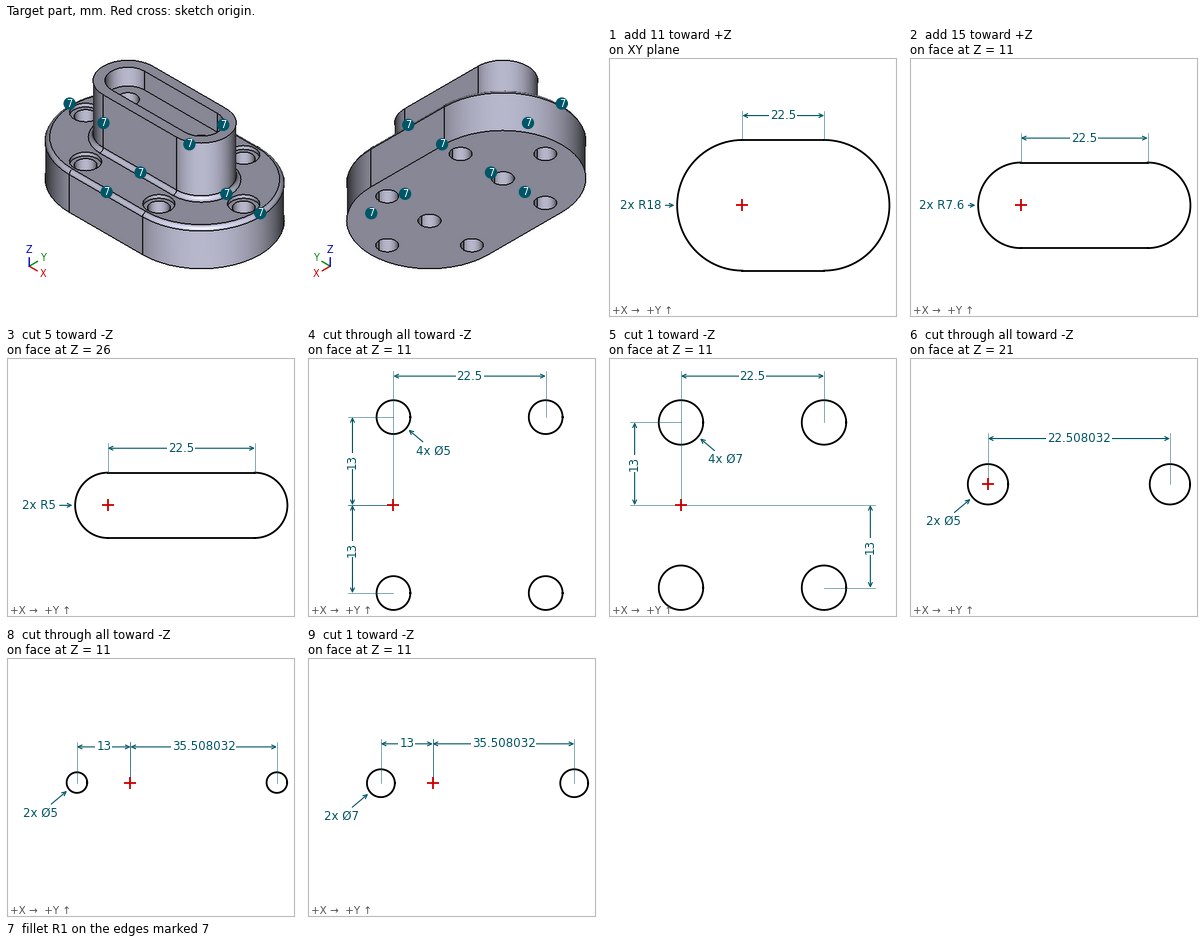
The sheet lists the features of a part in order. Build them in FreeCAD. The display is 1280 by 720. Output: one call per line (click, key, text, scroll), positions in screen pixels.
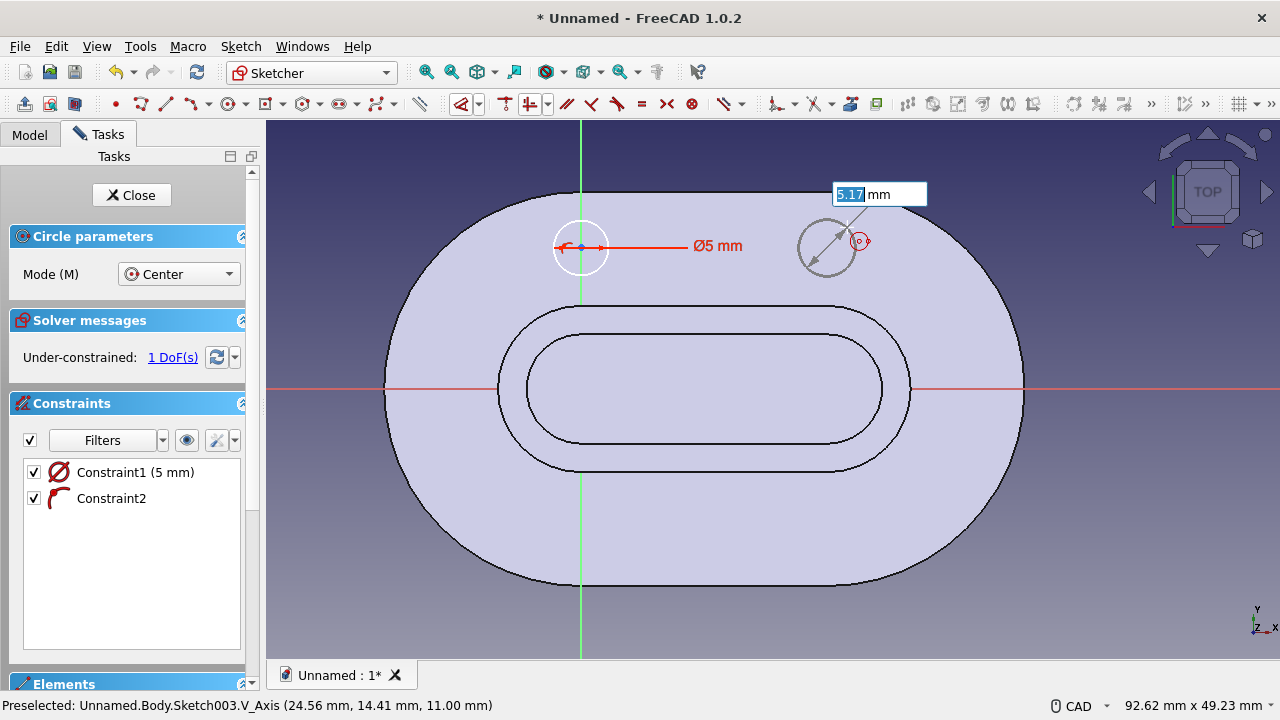
text(5)
key(Return)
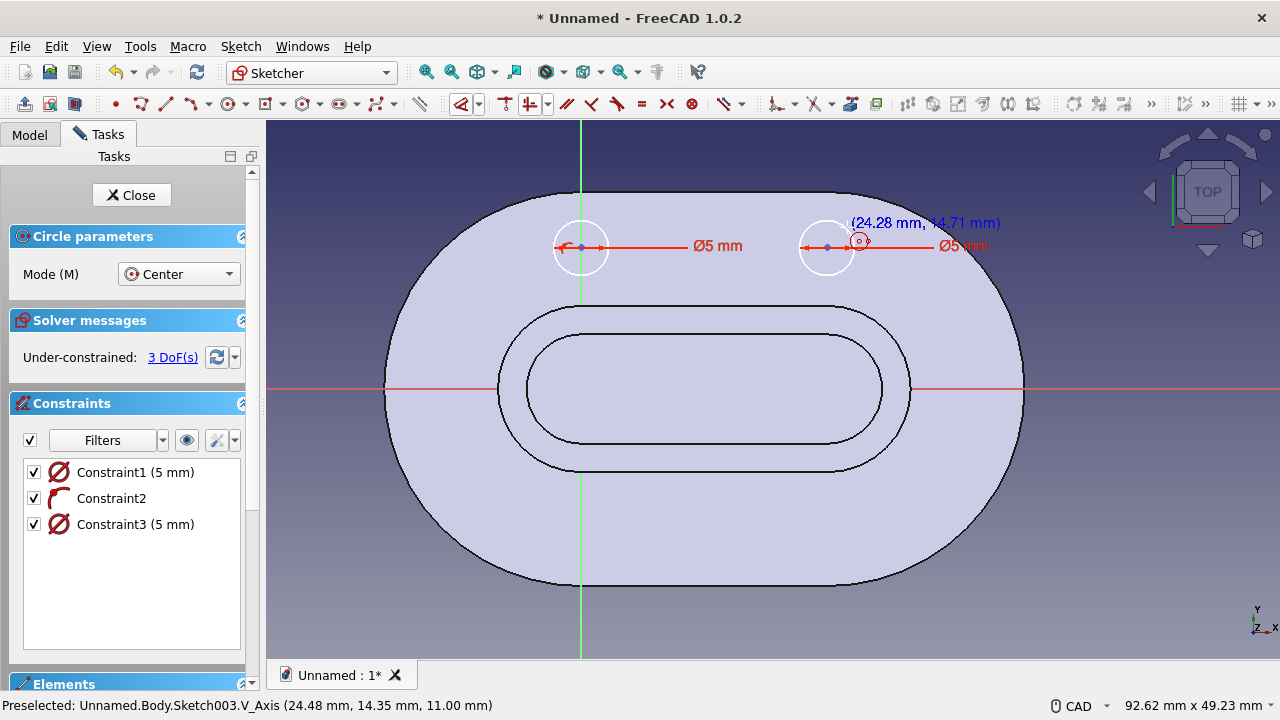
click(581, 531)
move(601, 512)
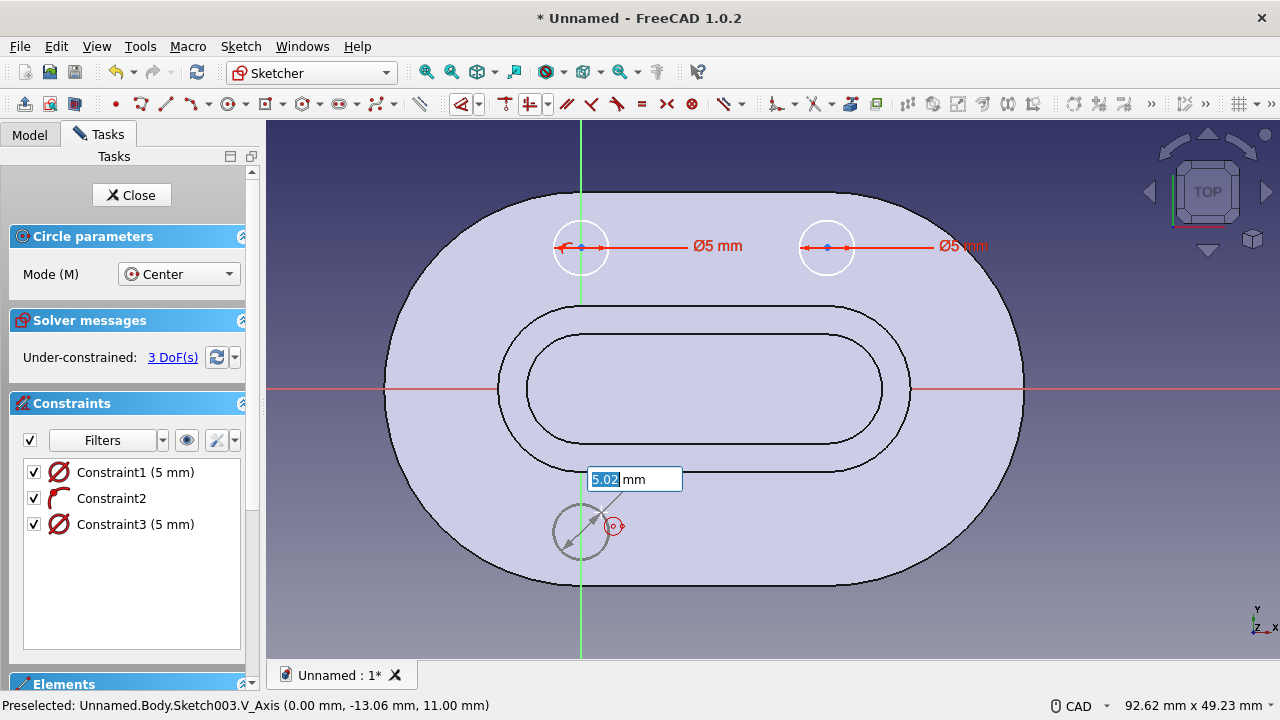
text(5)
key(Return)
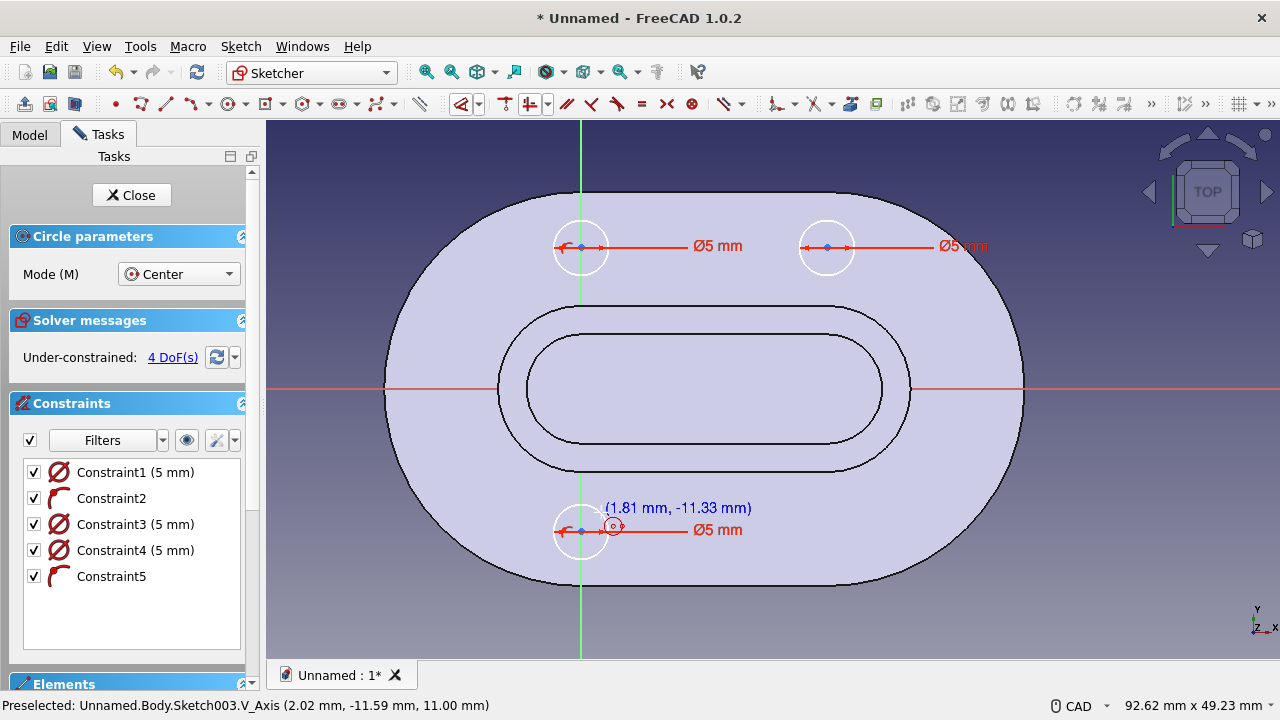
click(827, 531)
move(847, 512)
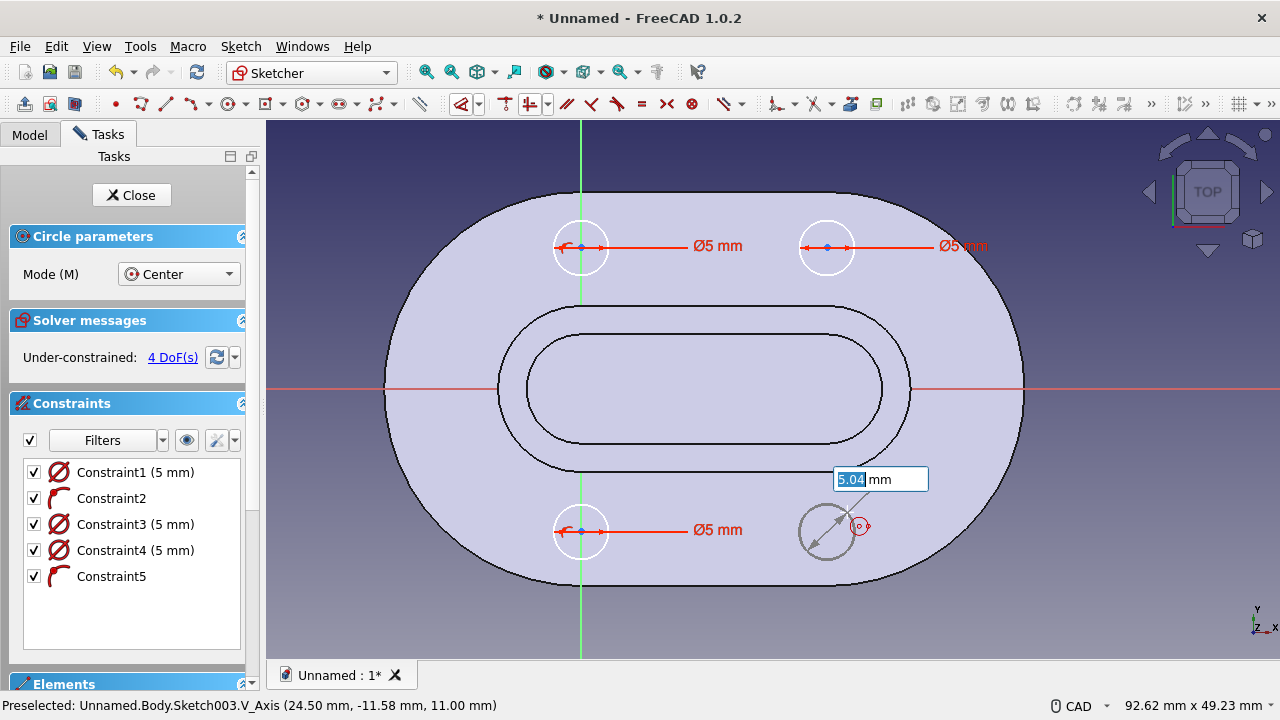
text(5)
key(Return)
key(Escape)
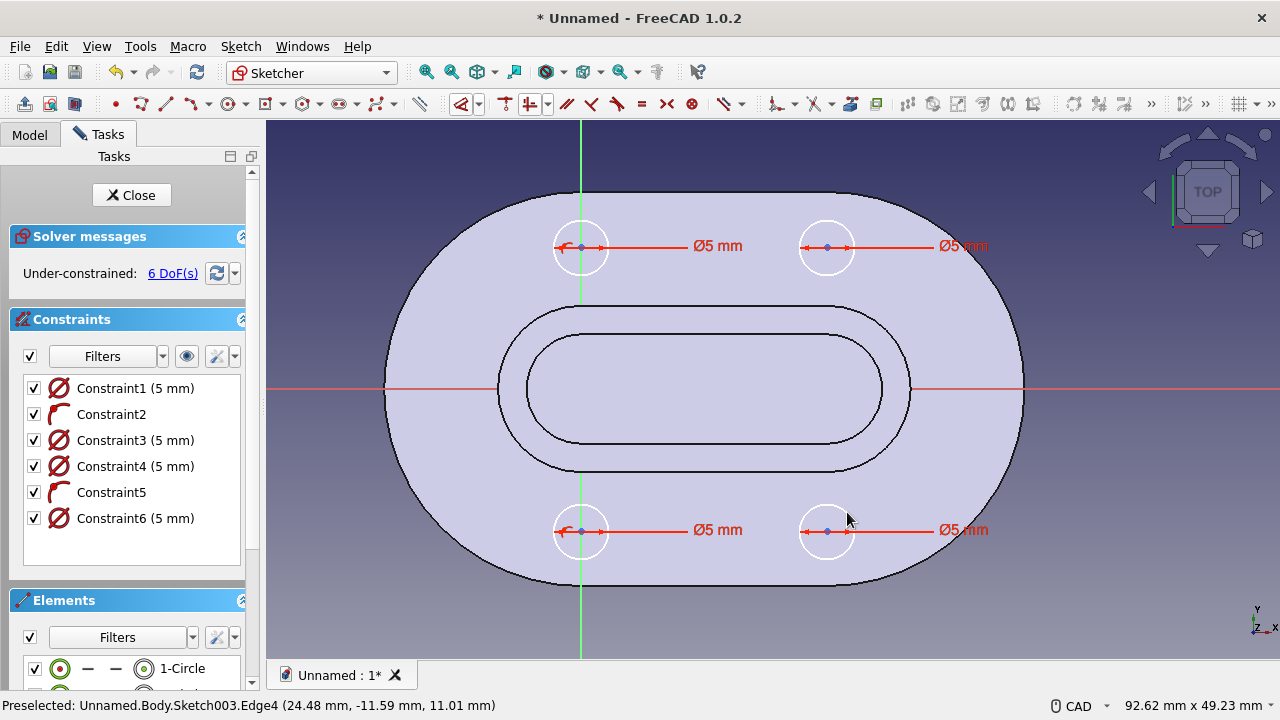
click(581, 248)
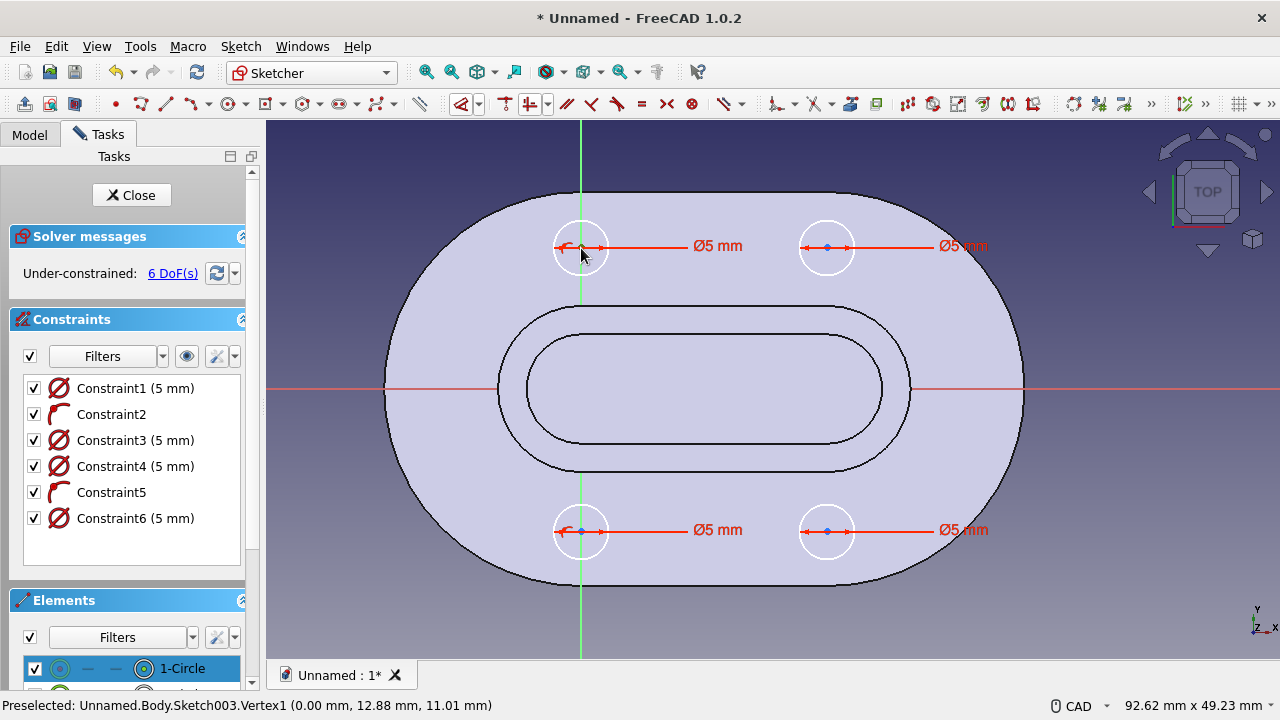
click(827, 248)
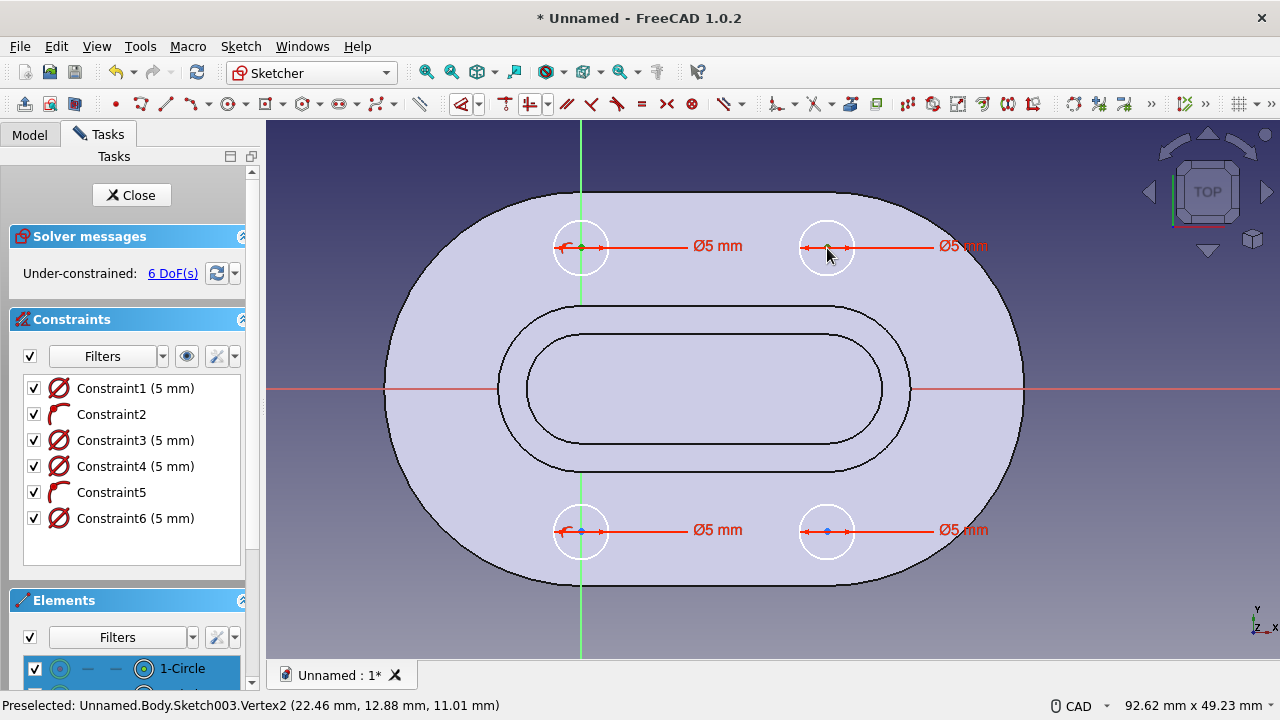
key(h)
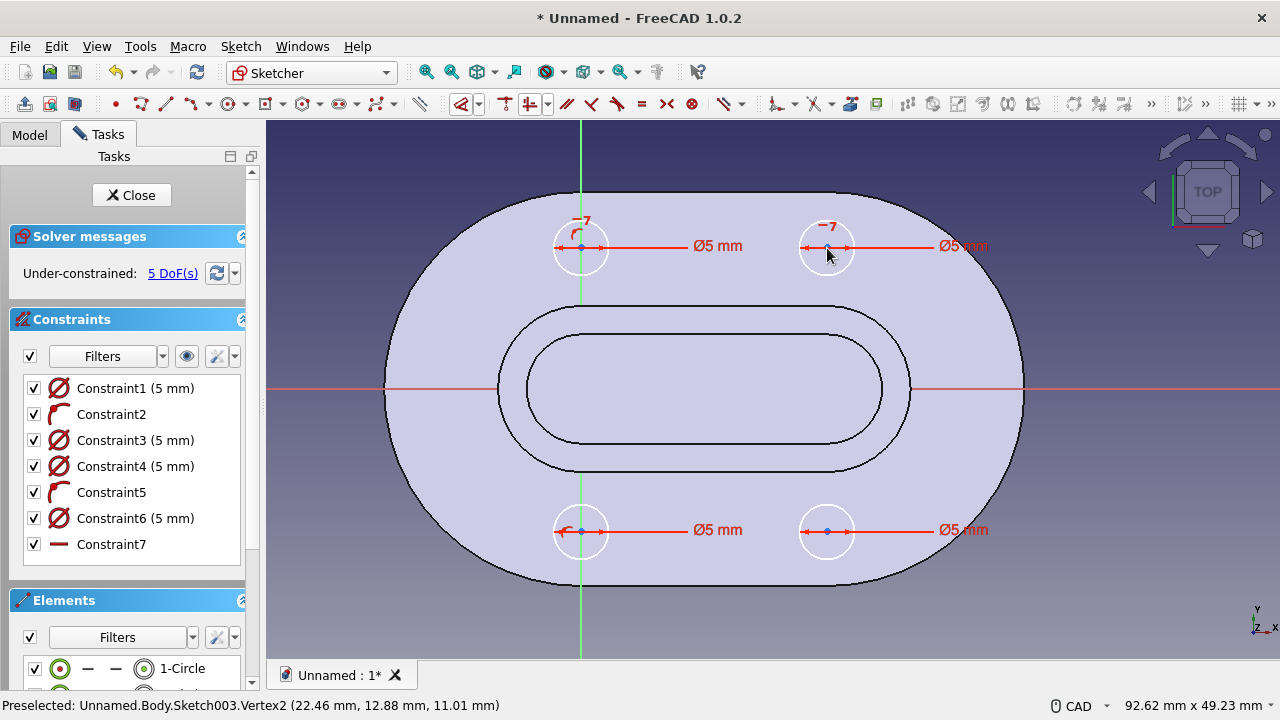
click(827, 248)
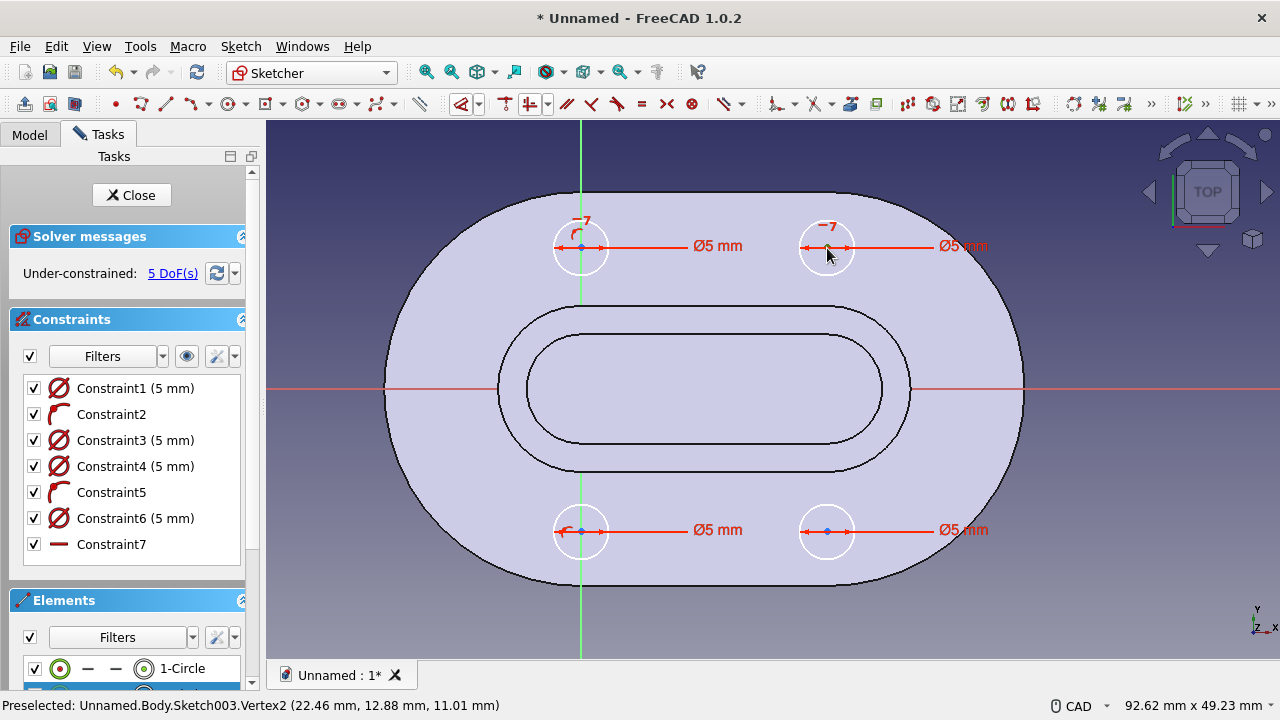
click(827, 532)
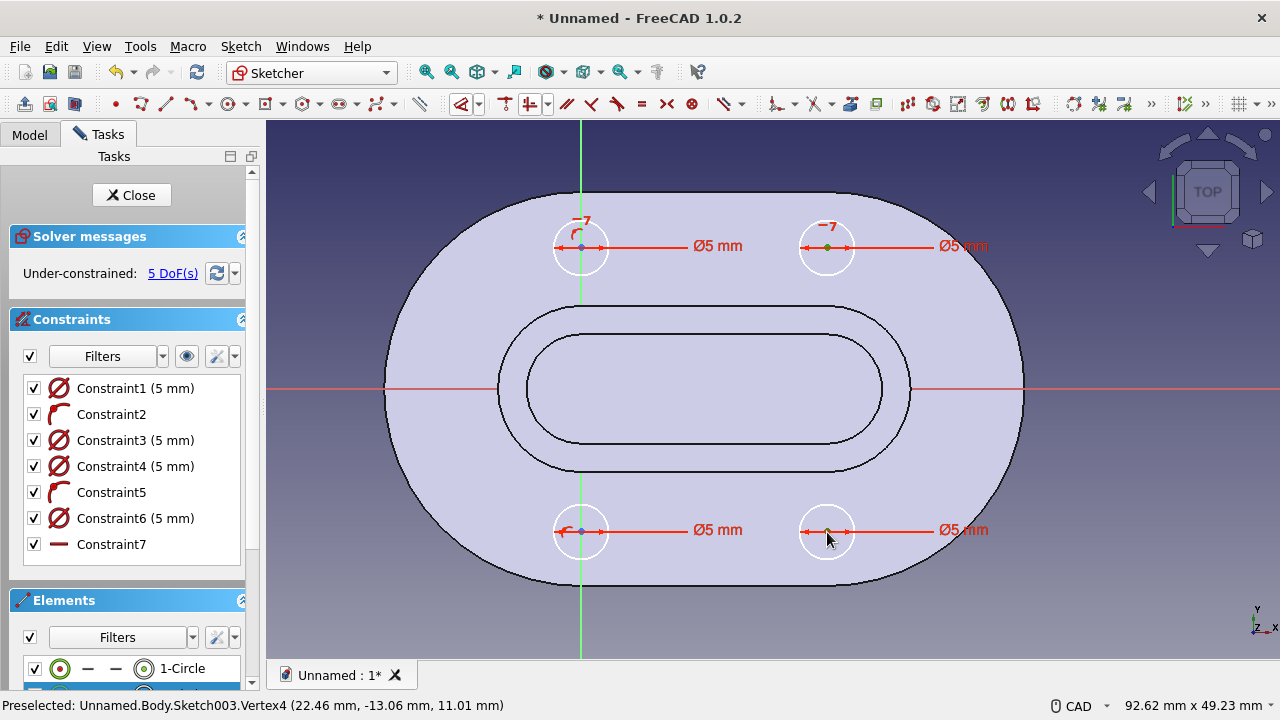
key(v)